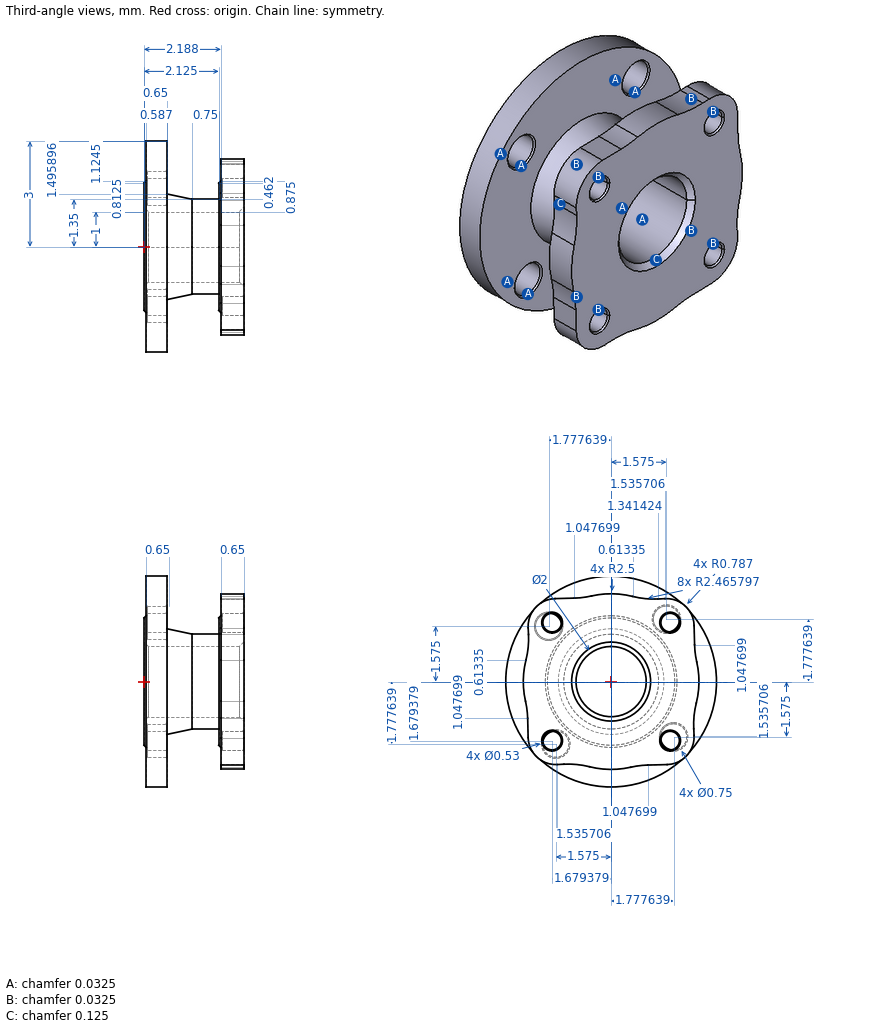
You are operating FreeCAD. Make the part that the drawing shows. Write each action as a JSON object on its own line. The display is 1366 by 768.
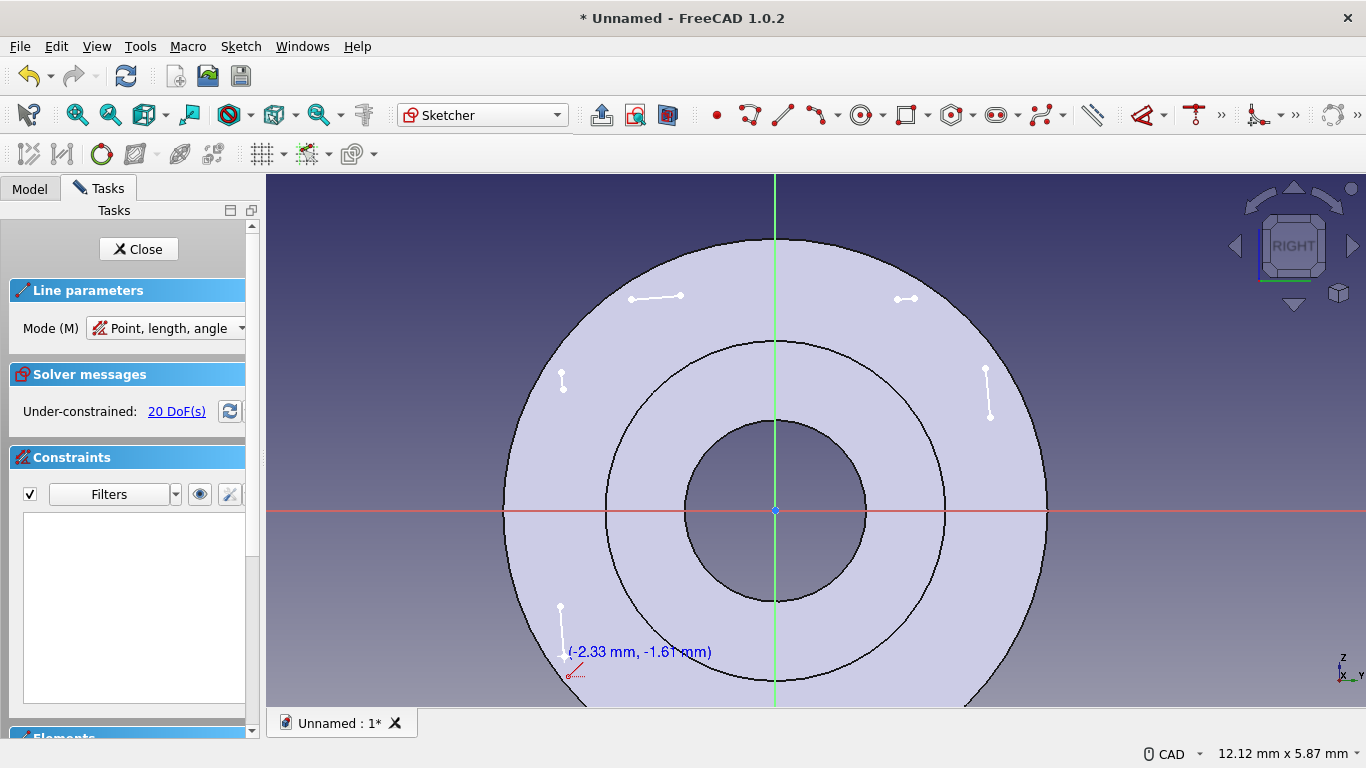
{"action": "scroll", "coordinate": [622, 202], "scroll_direction": "down", "scroll_amount": 1}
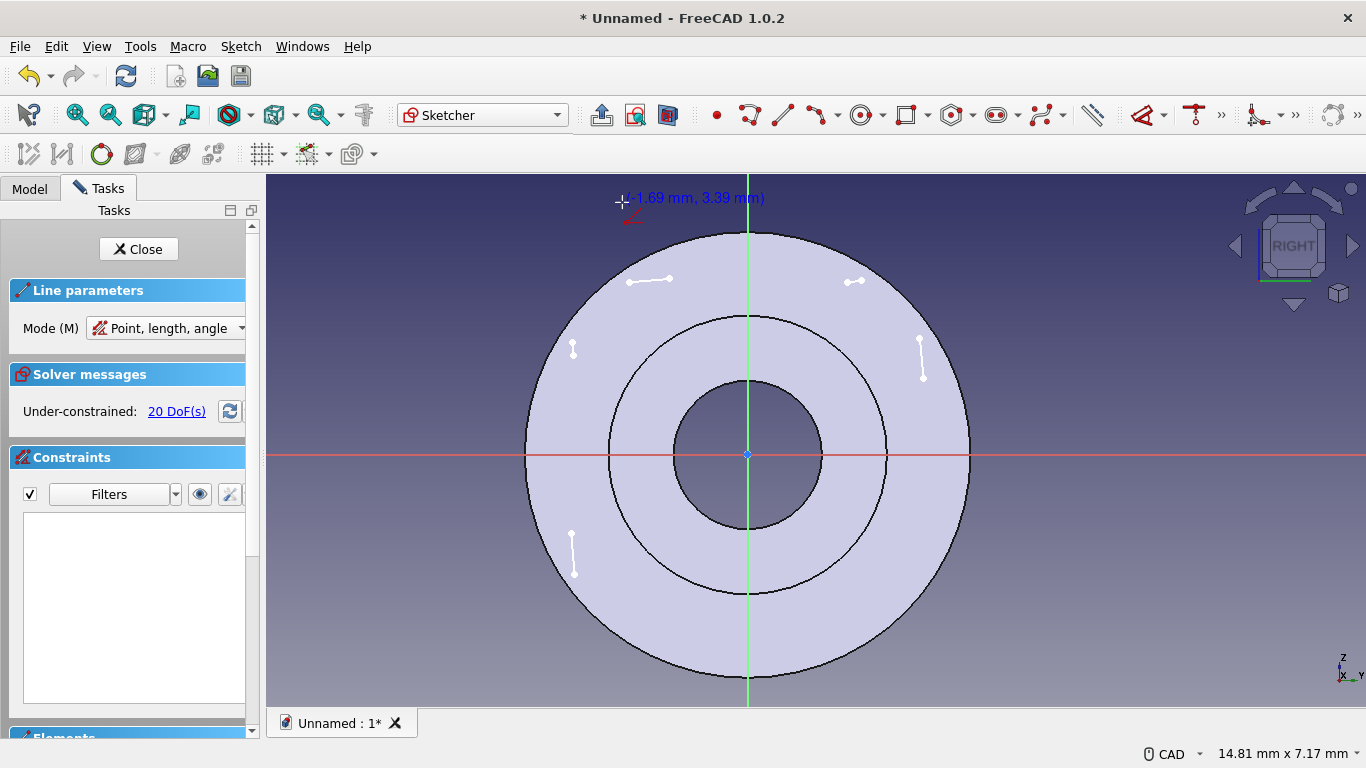
{"action": "left_click", "coordinate": [634, 630]}
{"action": "left_click", "coordinate": [648, 628]}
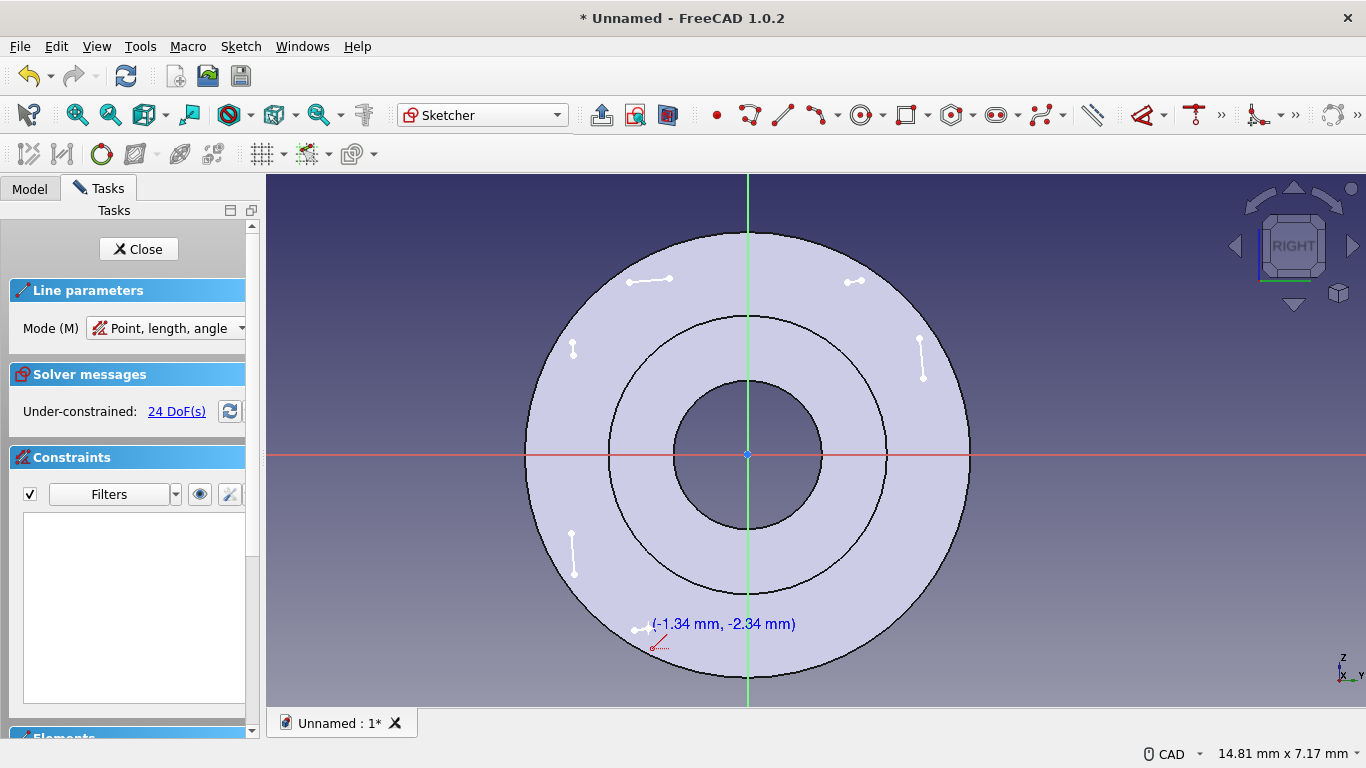
{"action": "left_click", "coordinate": [825, 631]}
{"action": "left_click", "coordinate": [866, 628]}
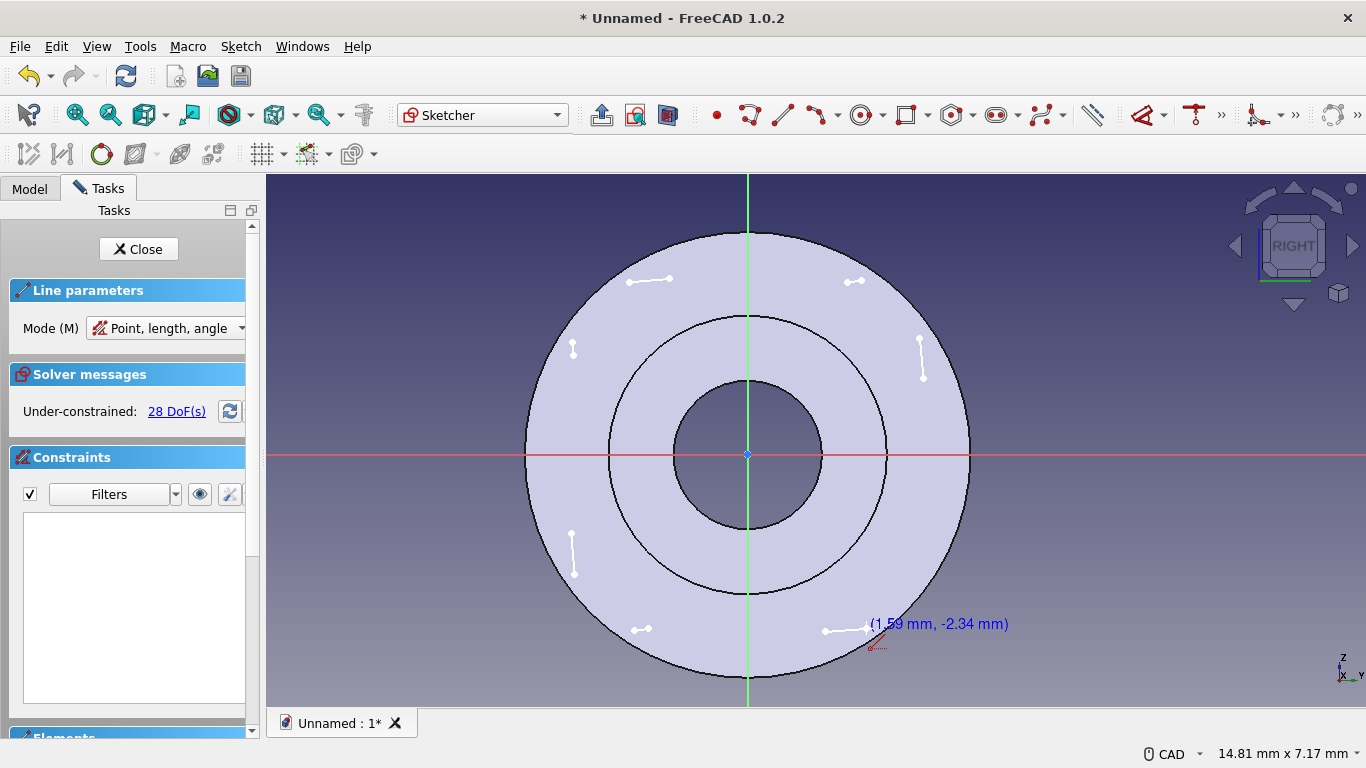
{"action": "left_click", "coordinate": [923, 569]}
{"action": "left_click", "coordinate": [921, 555]}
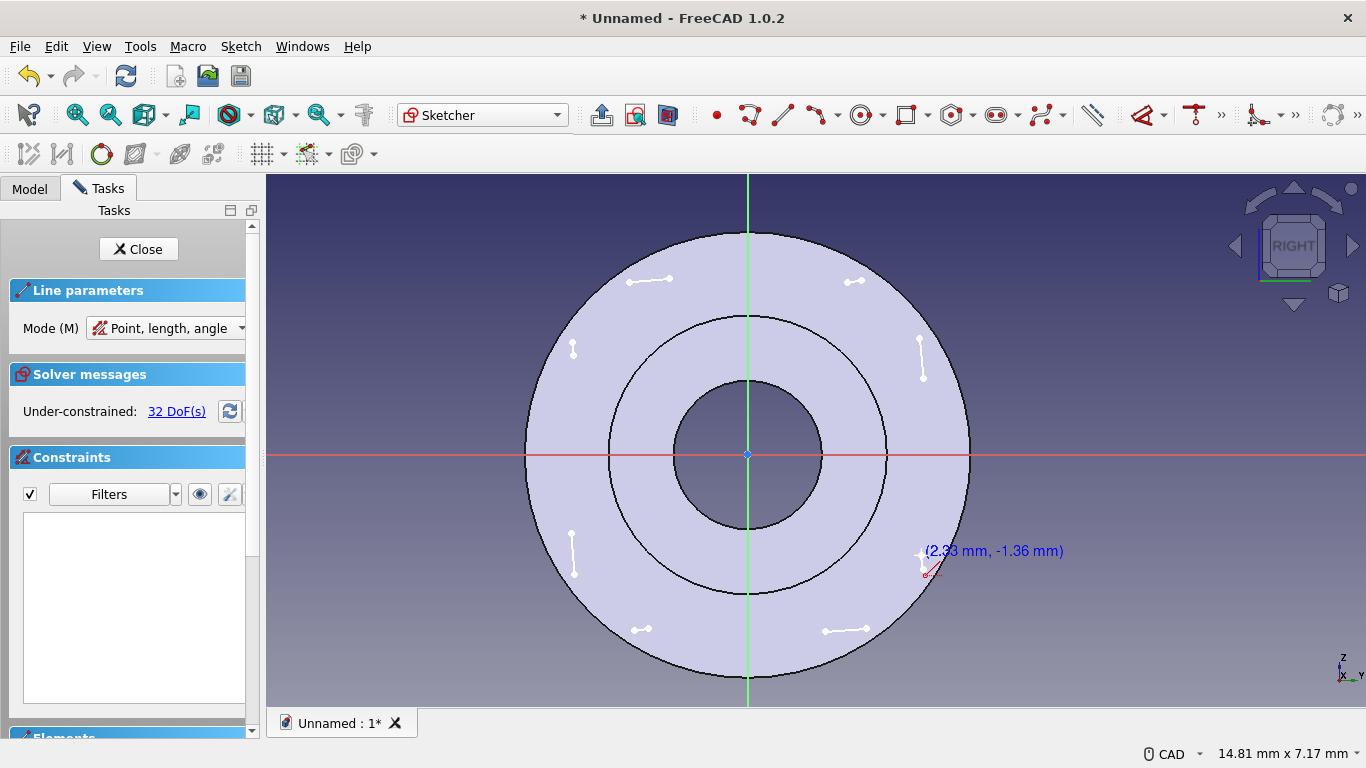
{"action": "left_click", "coordinate": [816, 116]}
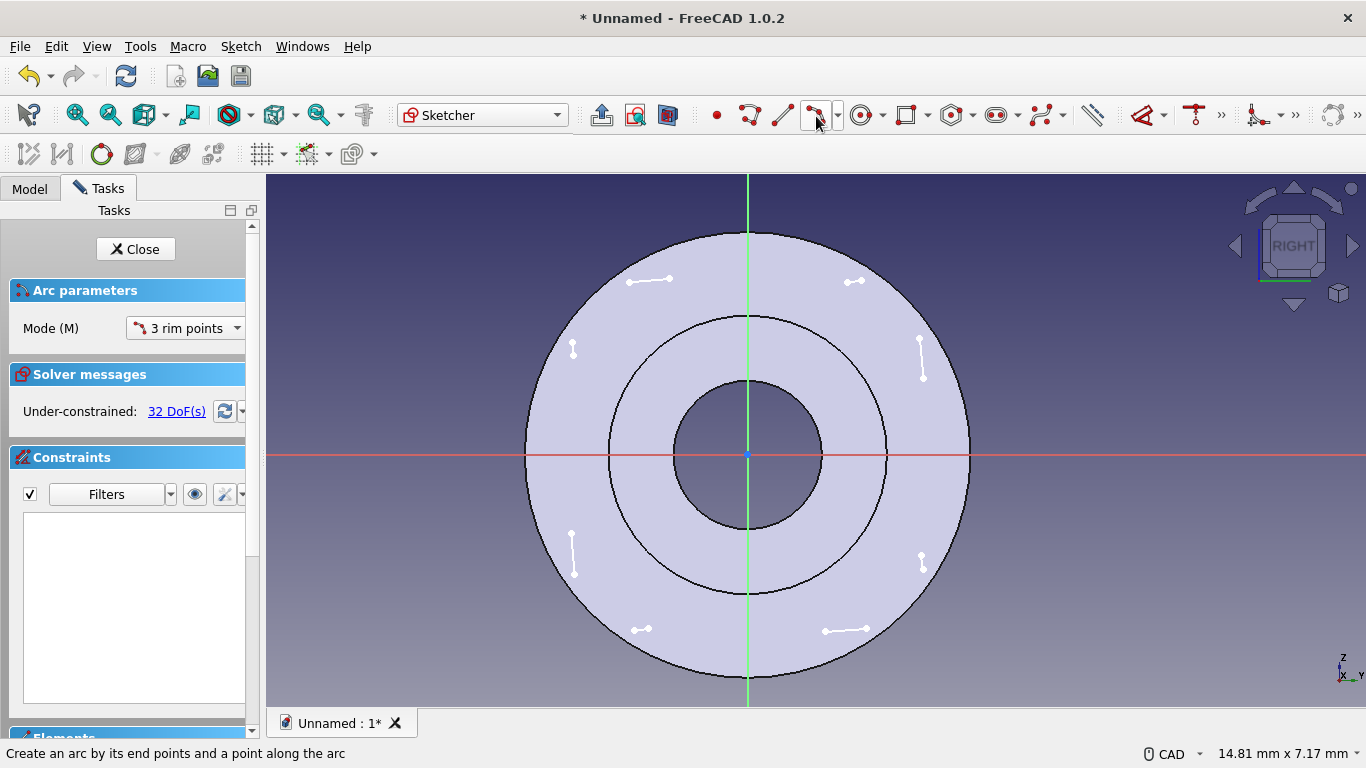
{"action": "left_click", "coordinate": [920, 338]}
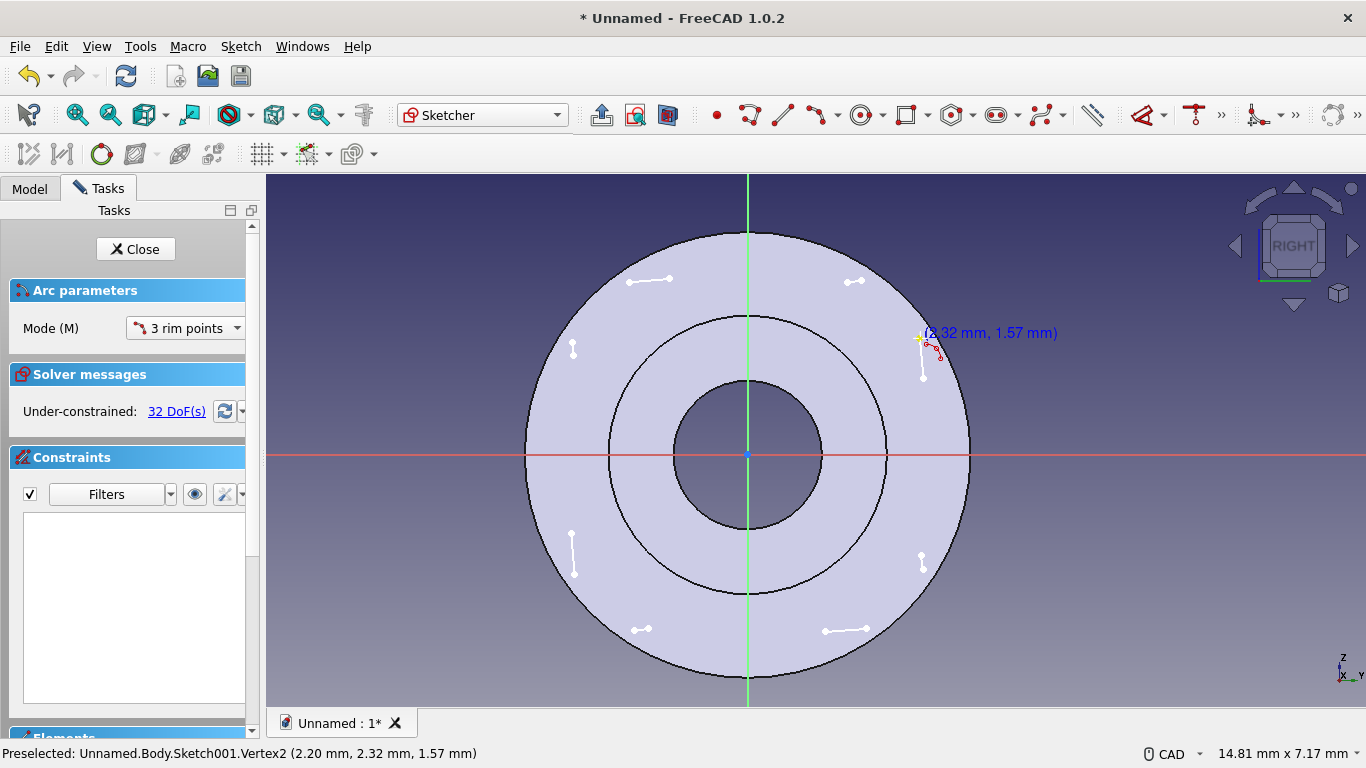
{"action": "scroll", "coordinate": [862, 280], "scroll_direction": "up", "scroll_amount": 4}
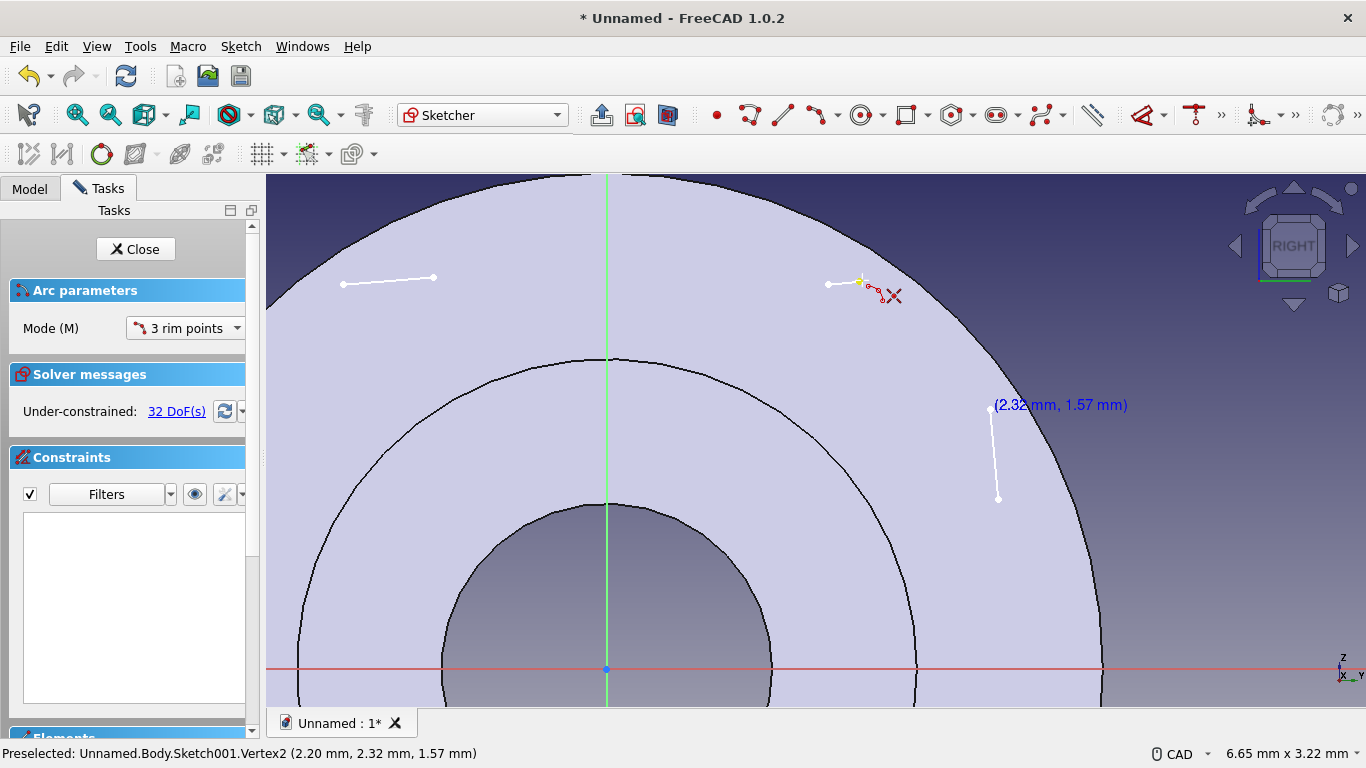
{"action": "left_click", "coordinate": [860, 282]}
{"action": "left_click", "coordinate": [956, 313]}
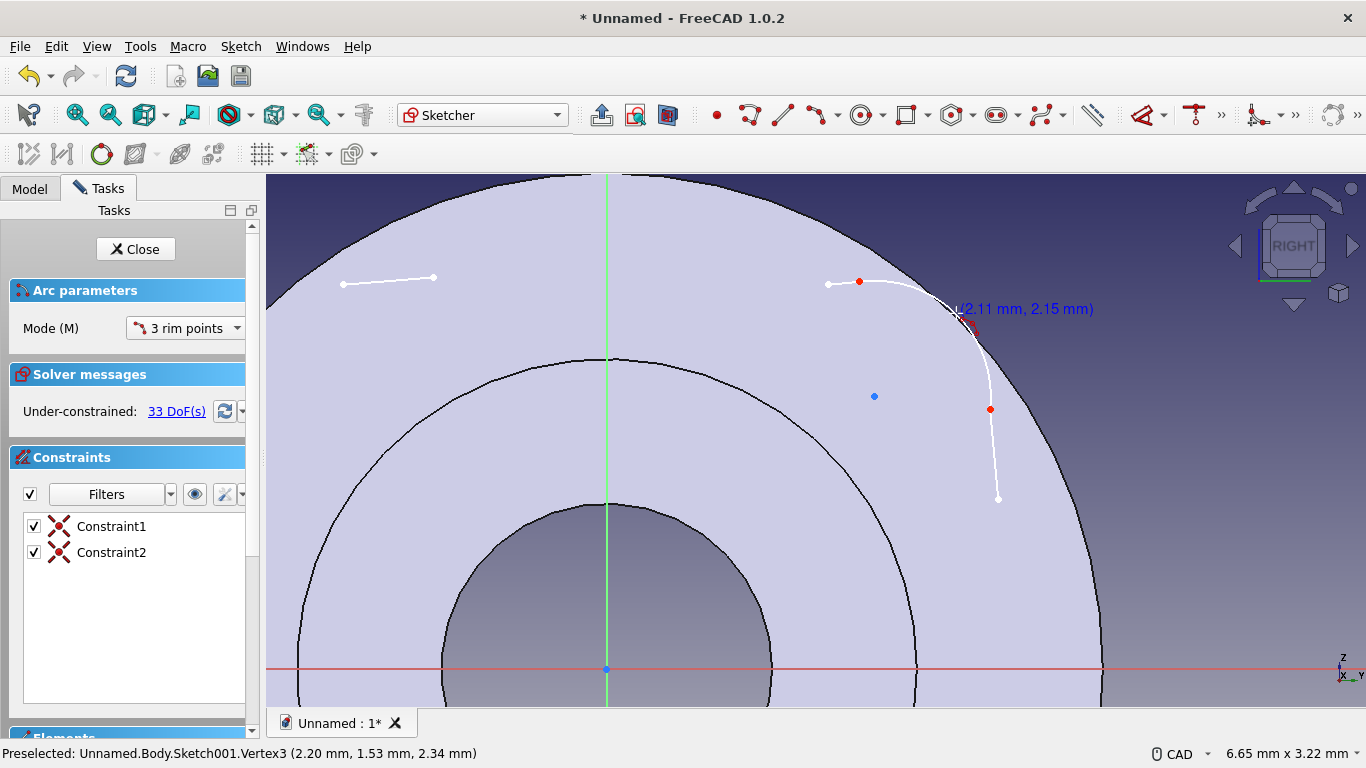
{"action": "left_click", "coordinate": [828, 285]}
{"action": "left_click", "coordinate": [708, 268]}